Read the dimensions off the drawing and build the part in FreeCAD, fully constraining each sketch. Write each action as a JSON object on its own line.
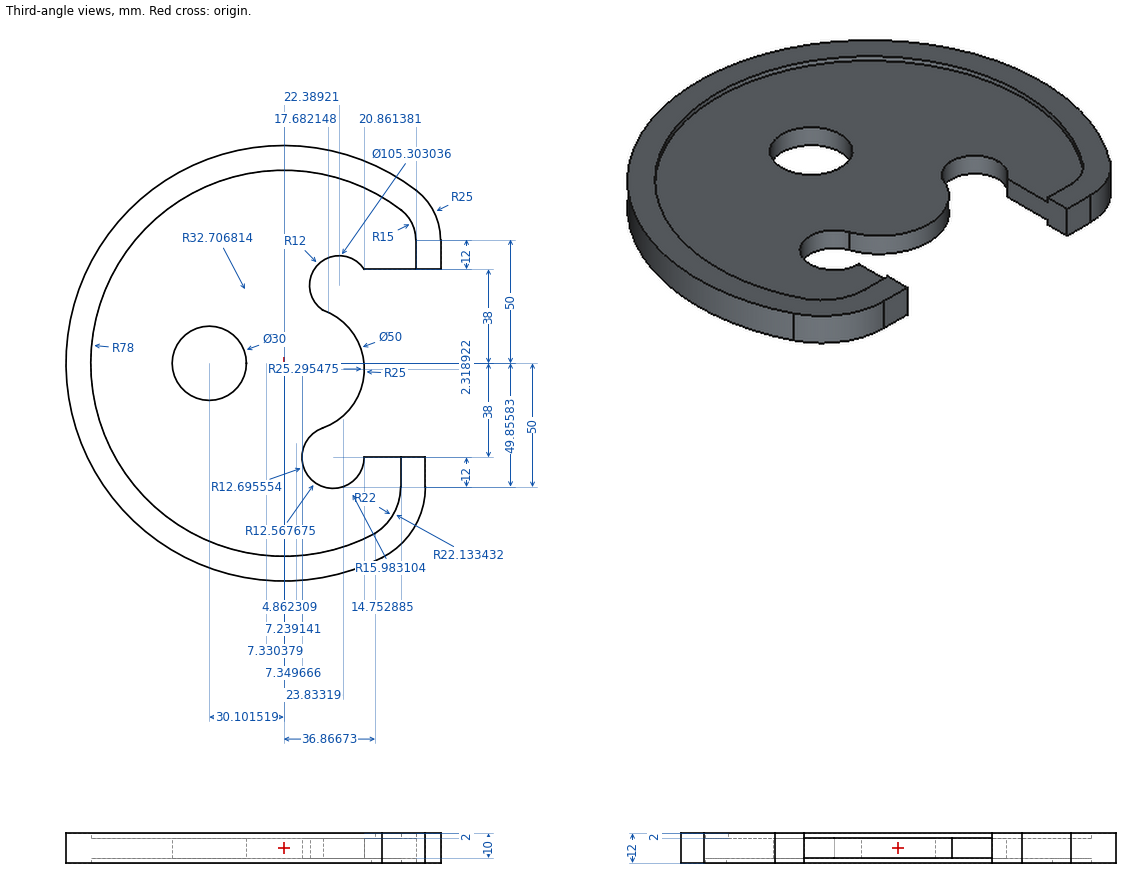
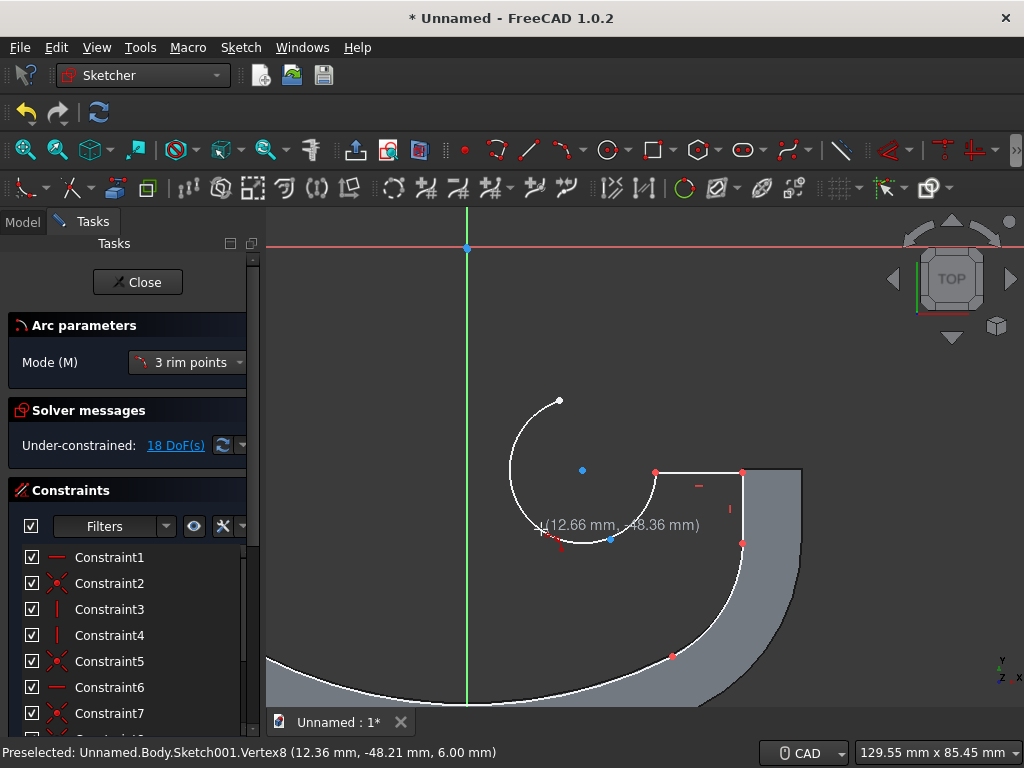
{"action": "left_click", "coordinate": [559, 401]}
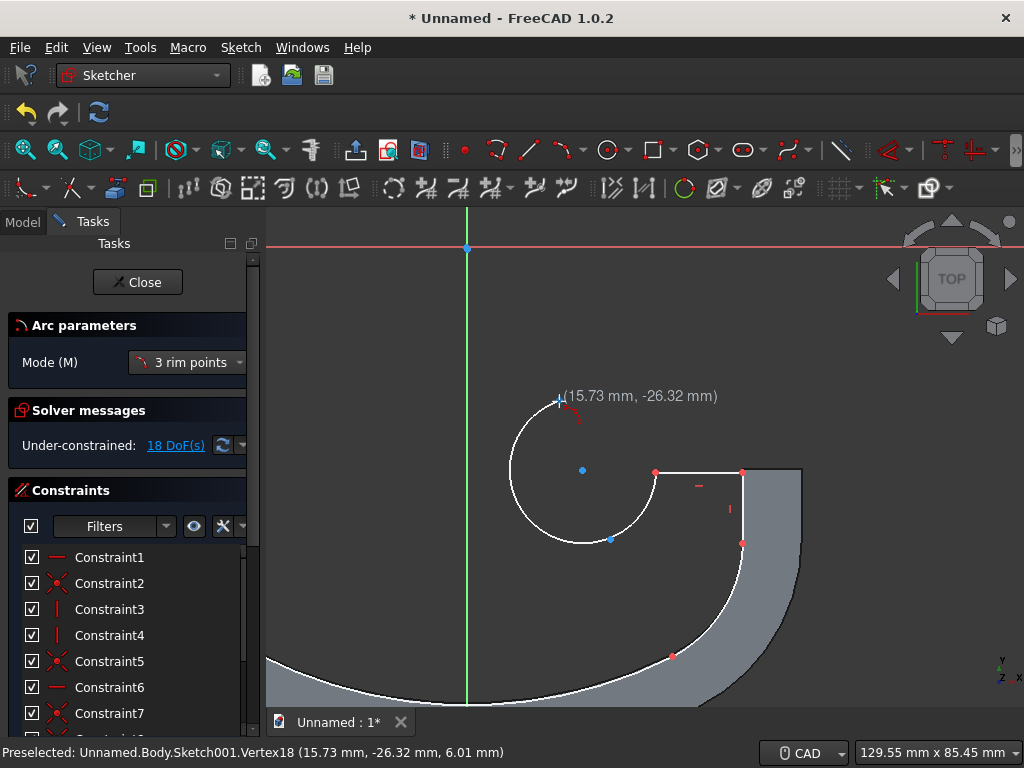
{"action": "scroll", "coordinate": [724, 610], "scroll_direction": "down", "scroll_amount": 4}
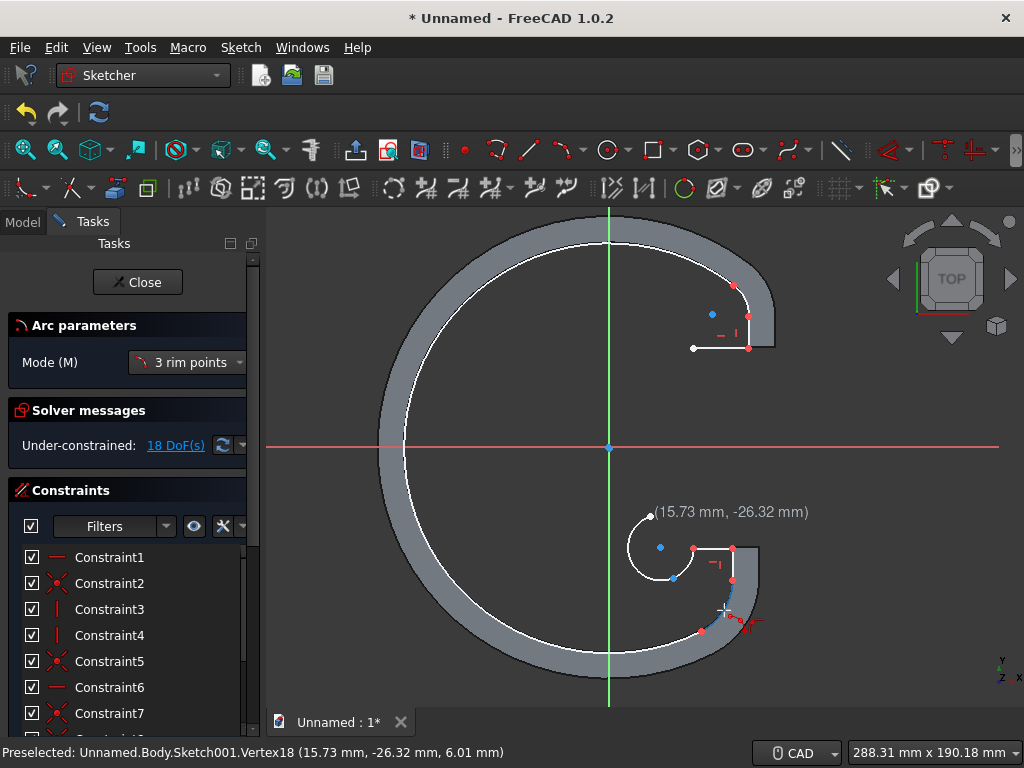
{"action": "left_click", "coordinate": [650, 391]}
{"action": "left_click", "coordinate": [692, 470]}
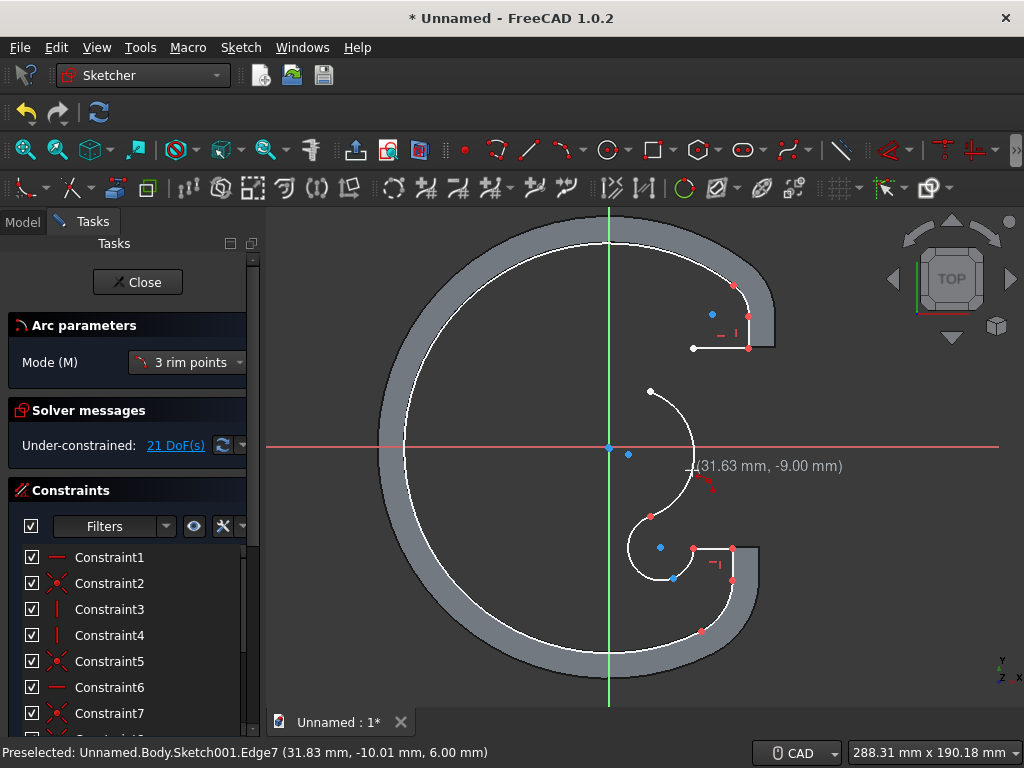
{"action": "left_click", "coordinate": [650, 392]}
{"action": "left_click", "coordinate": [694, 348]}
{"action": "left_click", "coordinate": [646, 342]}
{"action": "key", "text": "Escape"}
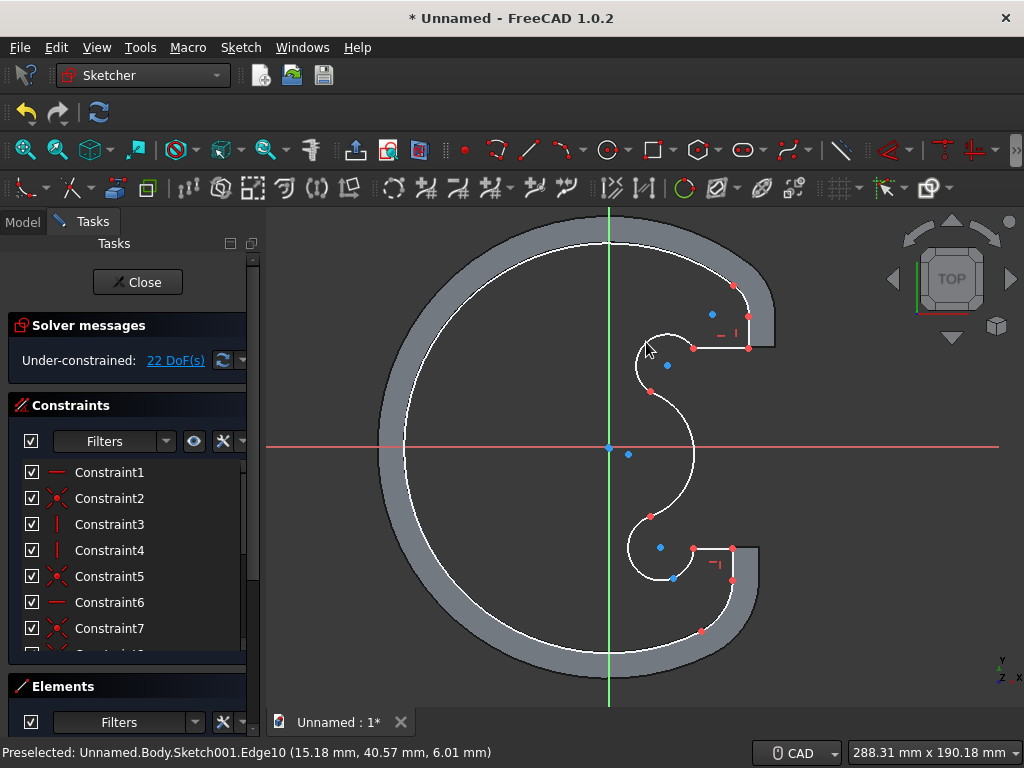
{"action": "scroll", "coordinate": [749, 339], "scroll_direction": "up", "scroll_amount": 2}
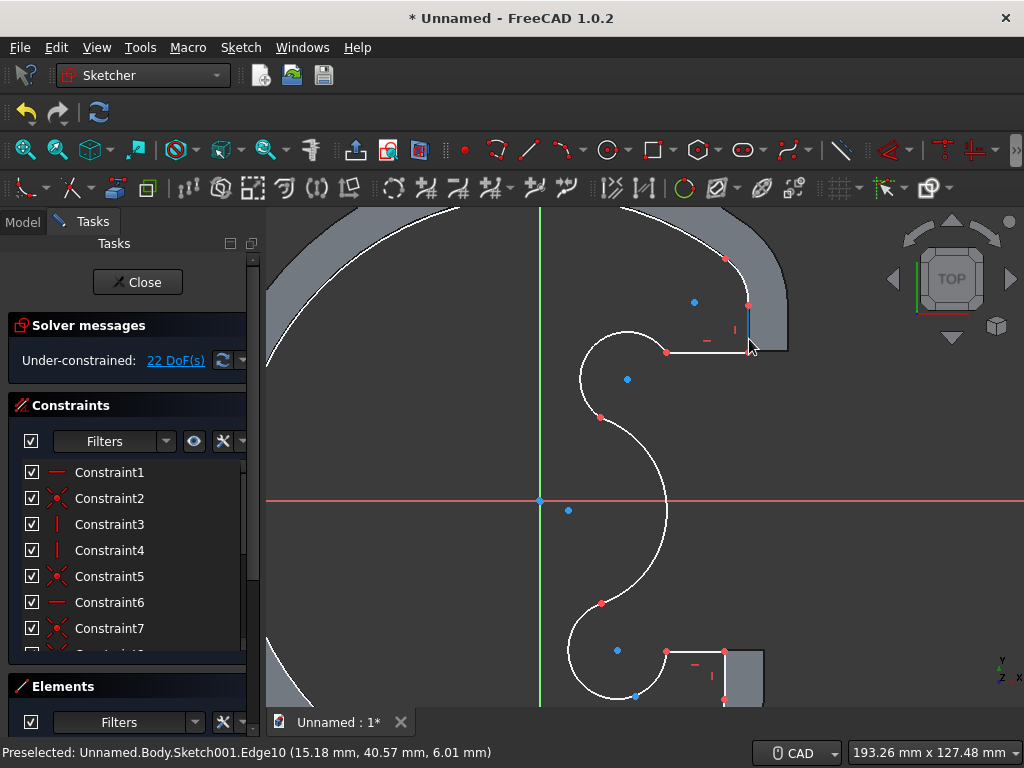
{"action": "left_click", "coordinate": [748, 339]}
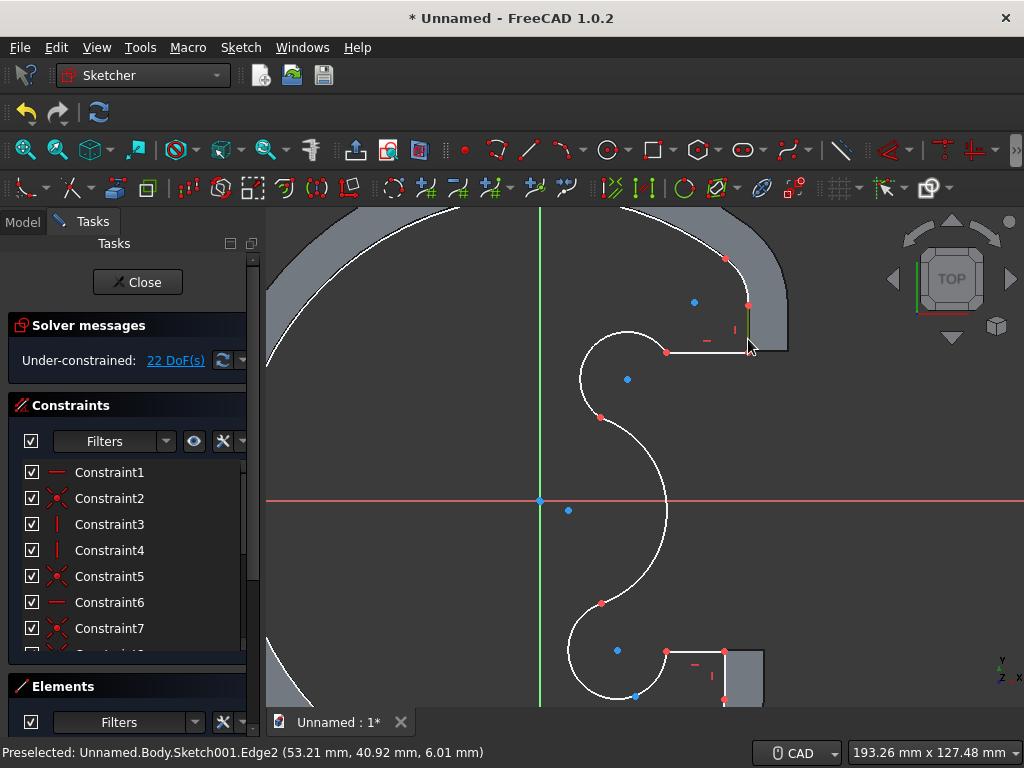
{"action": "left_click", "coordinate": [747, 289]}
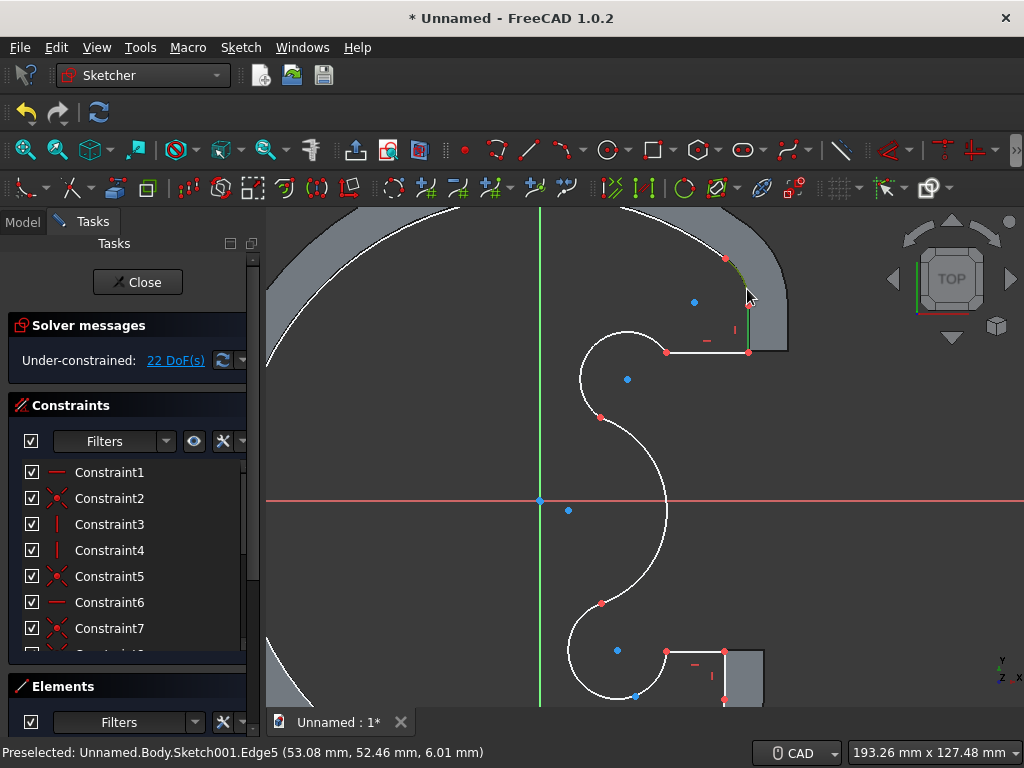
{"action": "key", "text": "t"}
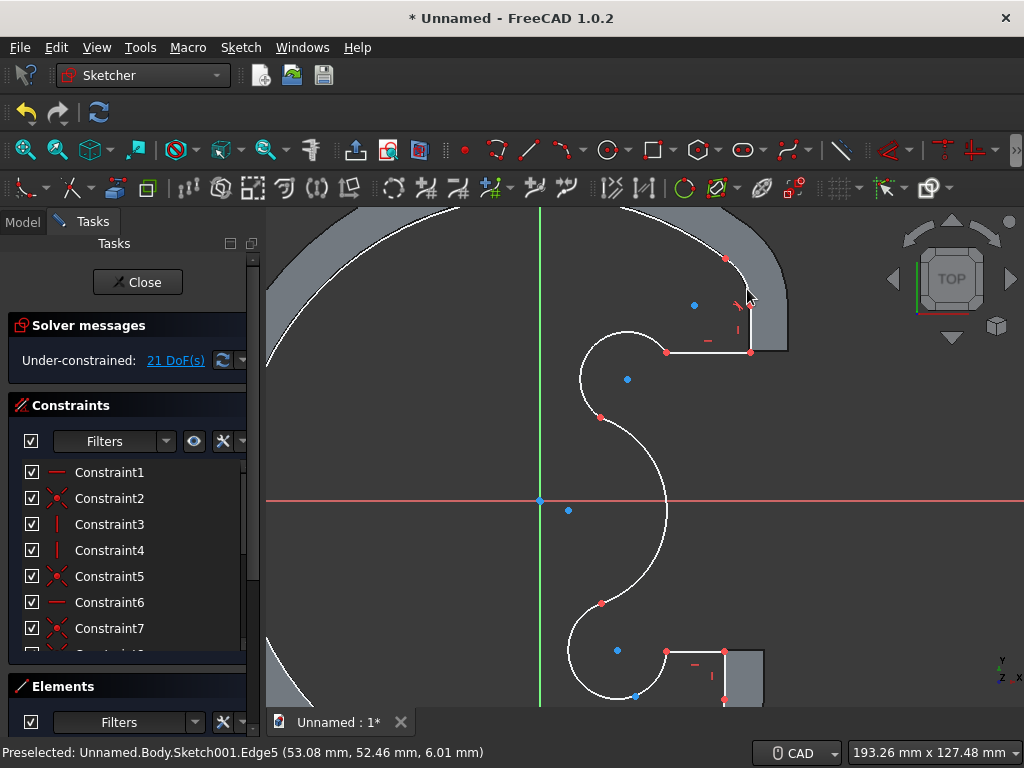
{"action": "left_click", "coordinate": [725, 666]}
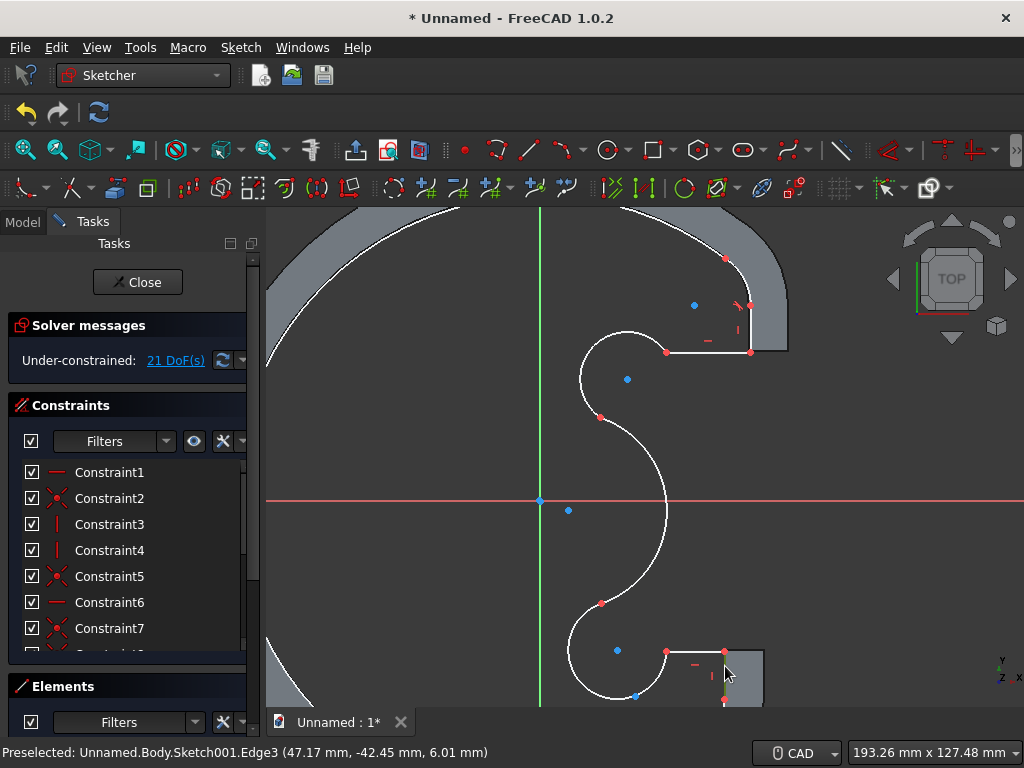
{"action": "scroll", "coordinate": [749, 338], "scroll_direction": "down", "scroll_amount": 2}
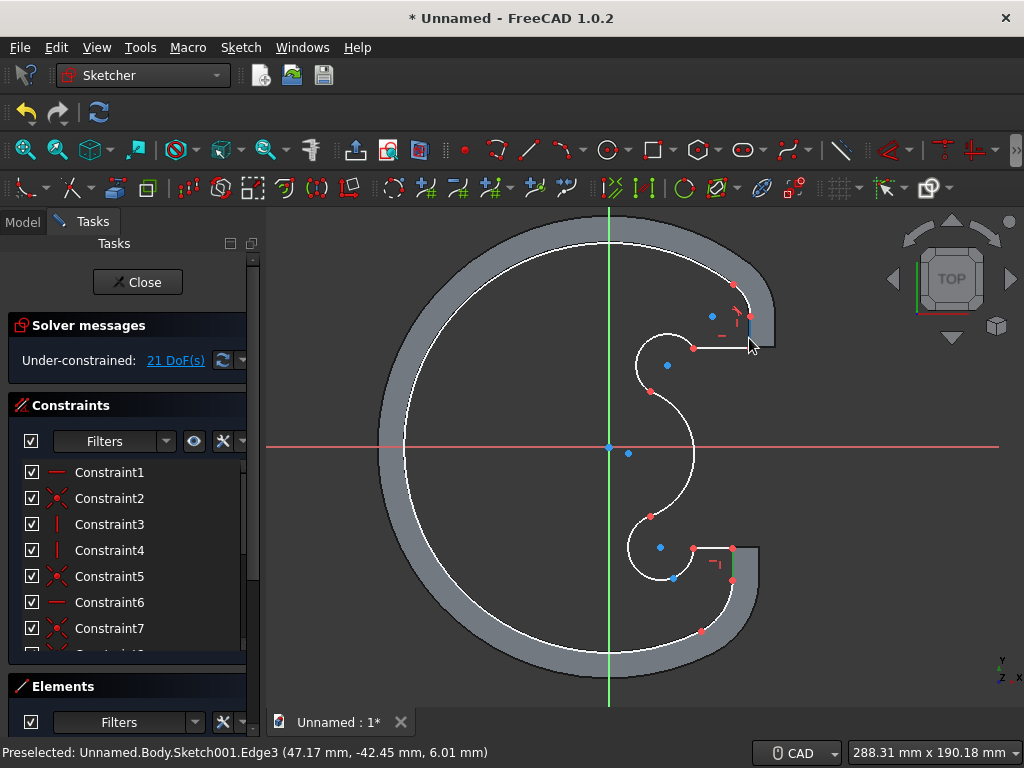
{"action": "left_click", "coordinate": [716, 620]}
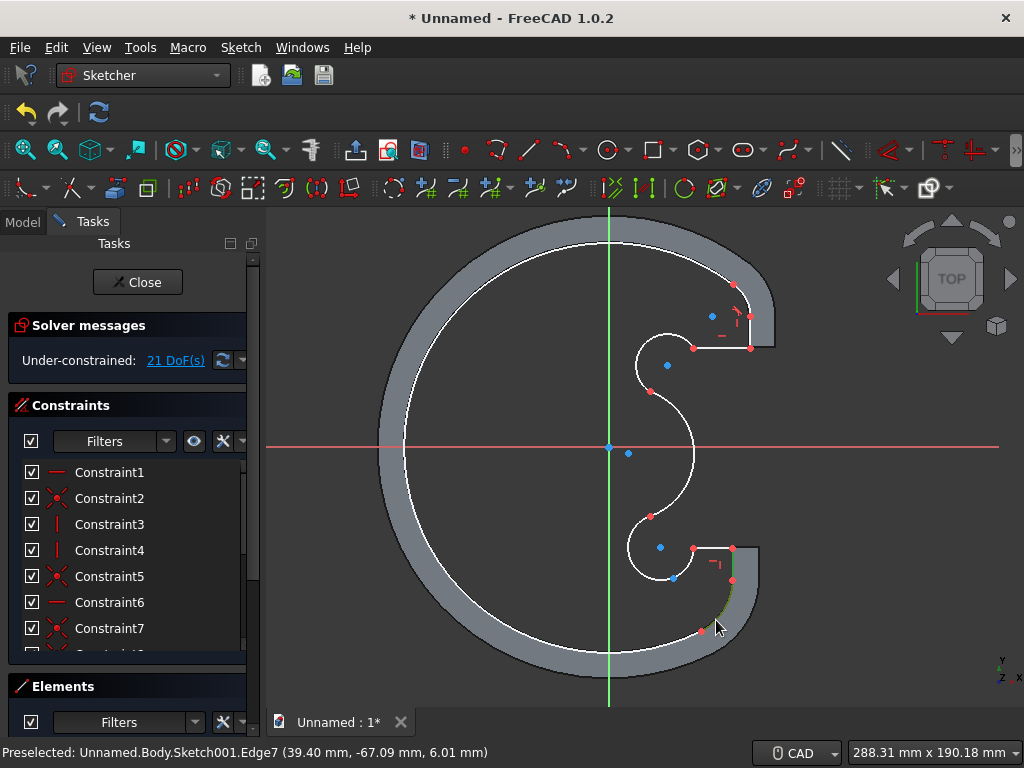
{"action": "key", "text": "t"}